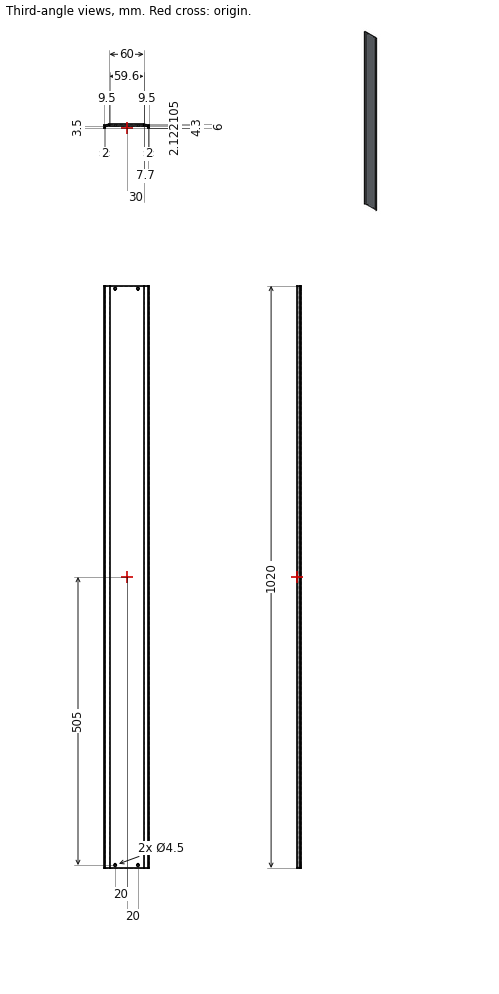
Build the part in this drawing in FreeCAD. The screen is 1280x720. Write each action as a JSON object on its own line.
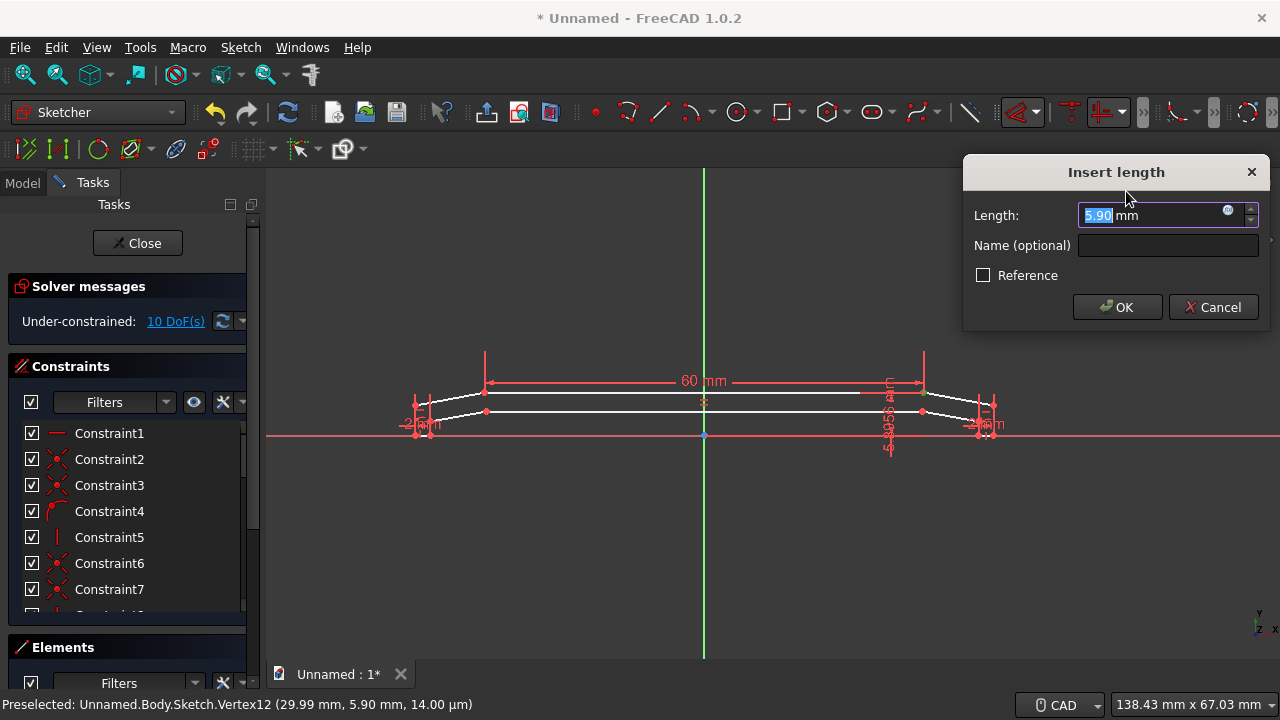
{"action": "type", "text": "6"}
{"action": "key", "text": "Return"}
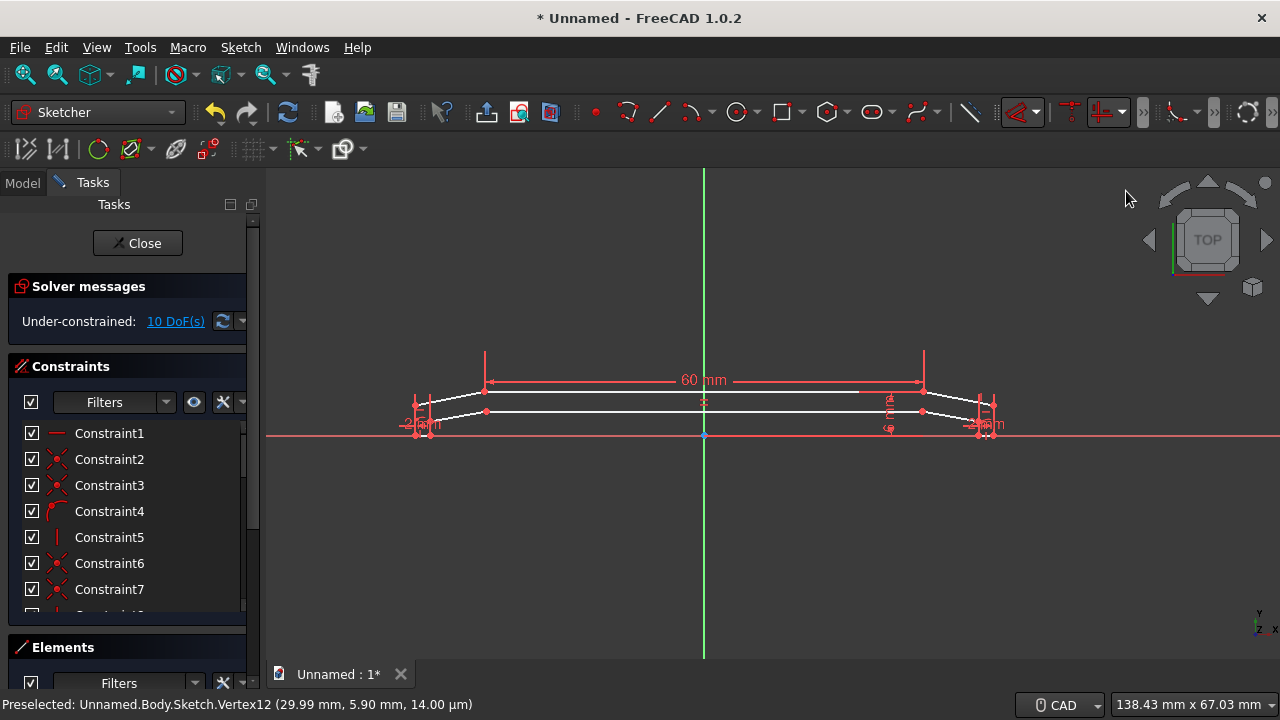
{"action": "scroll", "coordinate": [994, 427], "scroll_direction": "up", "scroll_amount": 3}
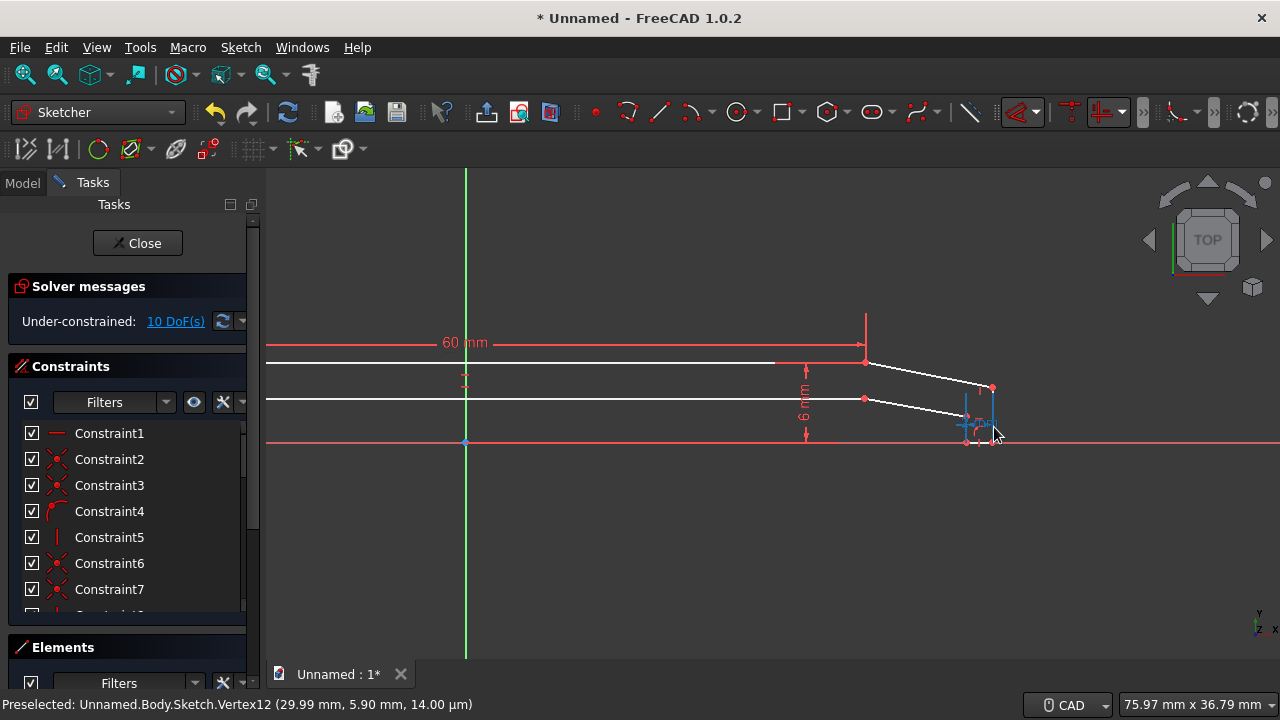
{"action": "left_click", "coordinate": [993, 404]}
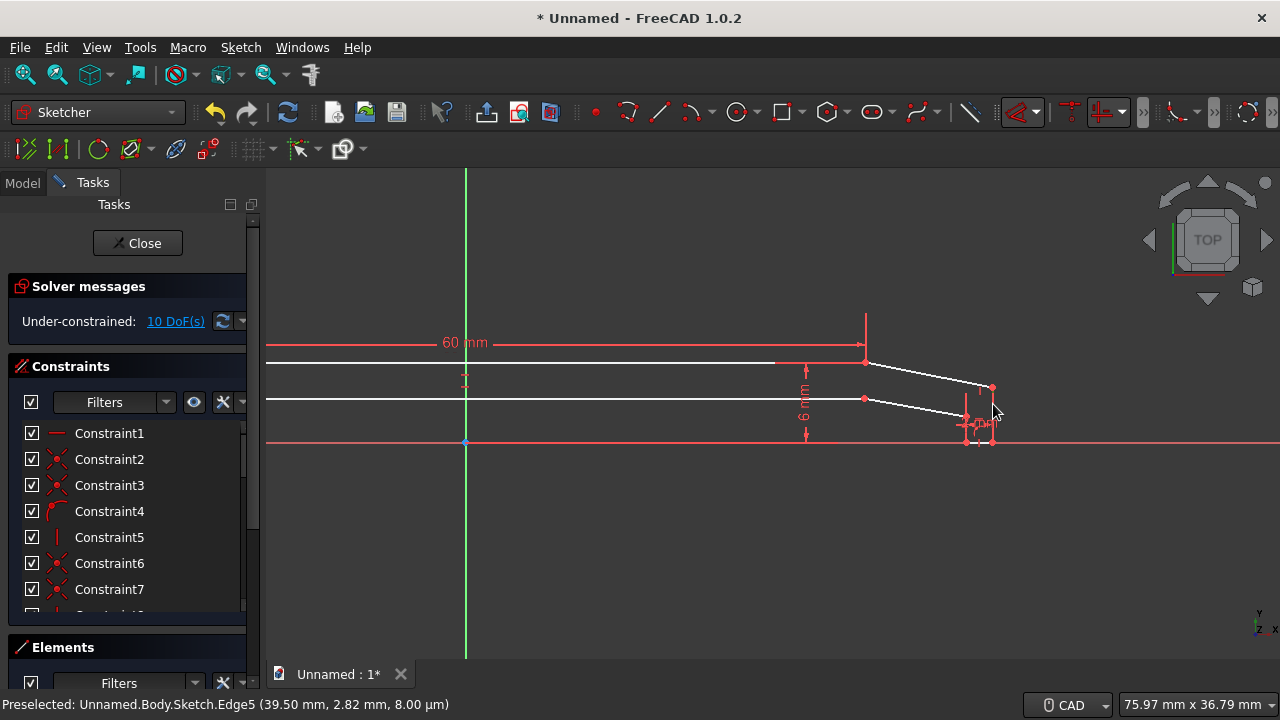
{"action": "left_click", "coordinate": [1038, 112]}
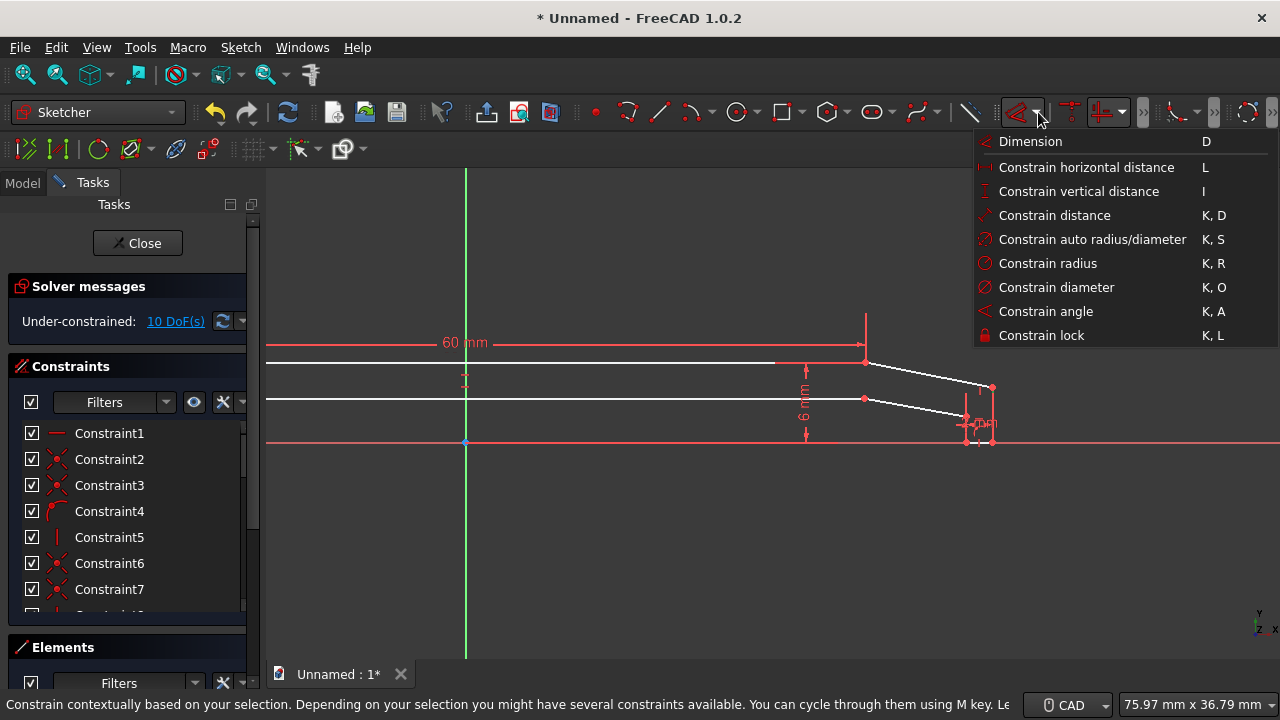
{"action": "left_click", "coordinate": [1126, 191]}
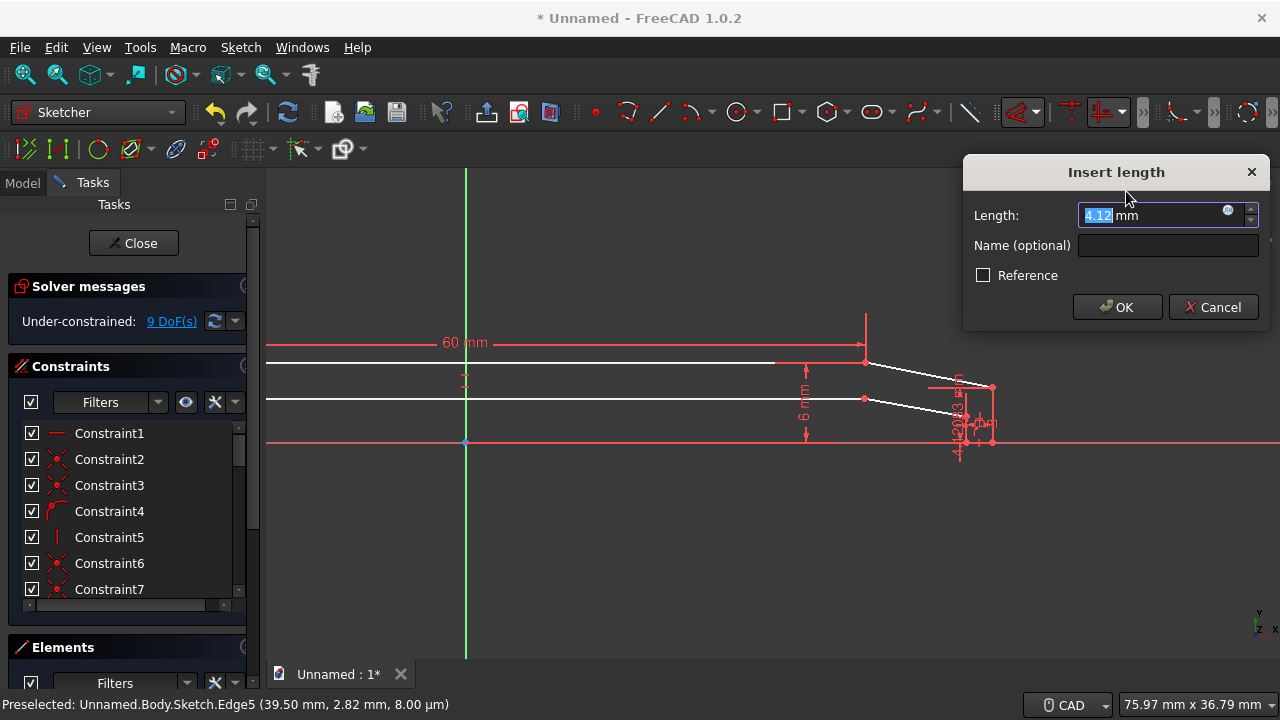
{"action": "type", "text": "4.3"}
{"action": "key", "text": "Return"}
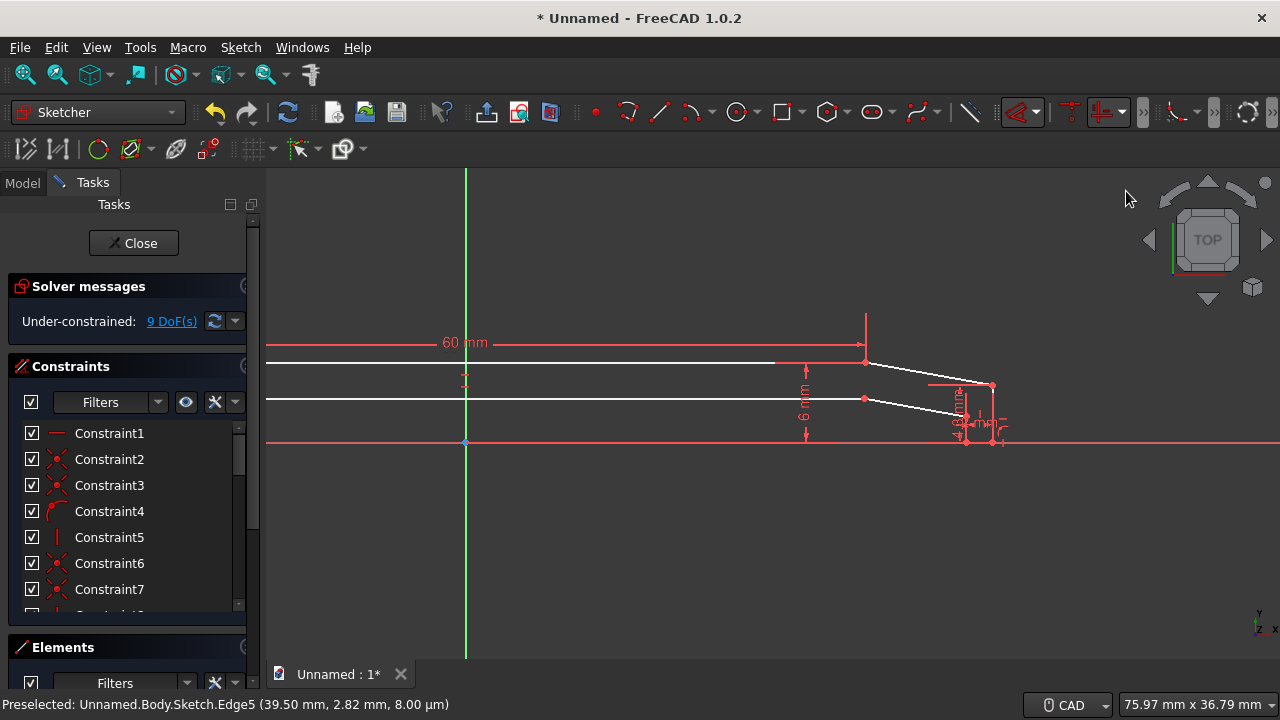
{"action": "scroll", "coordinate": [995, 427], "scroll_direction": "down", "scroll_amount": 3}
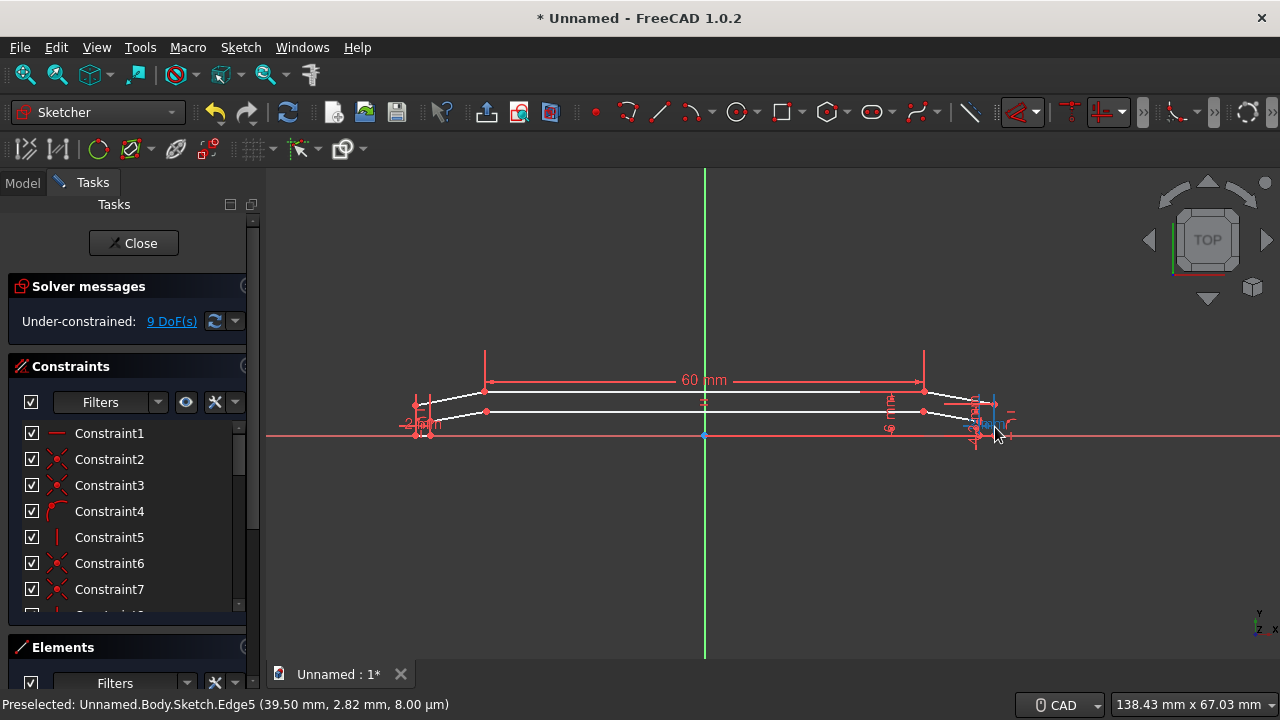
{"action": "scroll", "coordinate": [416, 415], "scroll_direction": "up", "scroll_amount": 3}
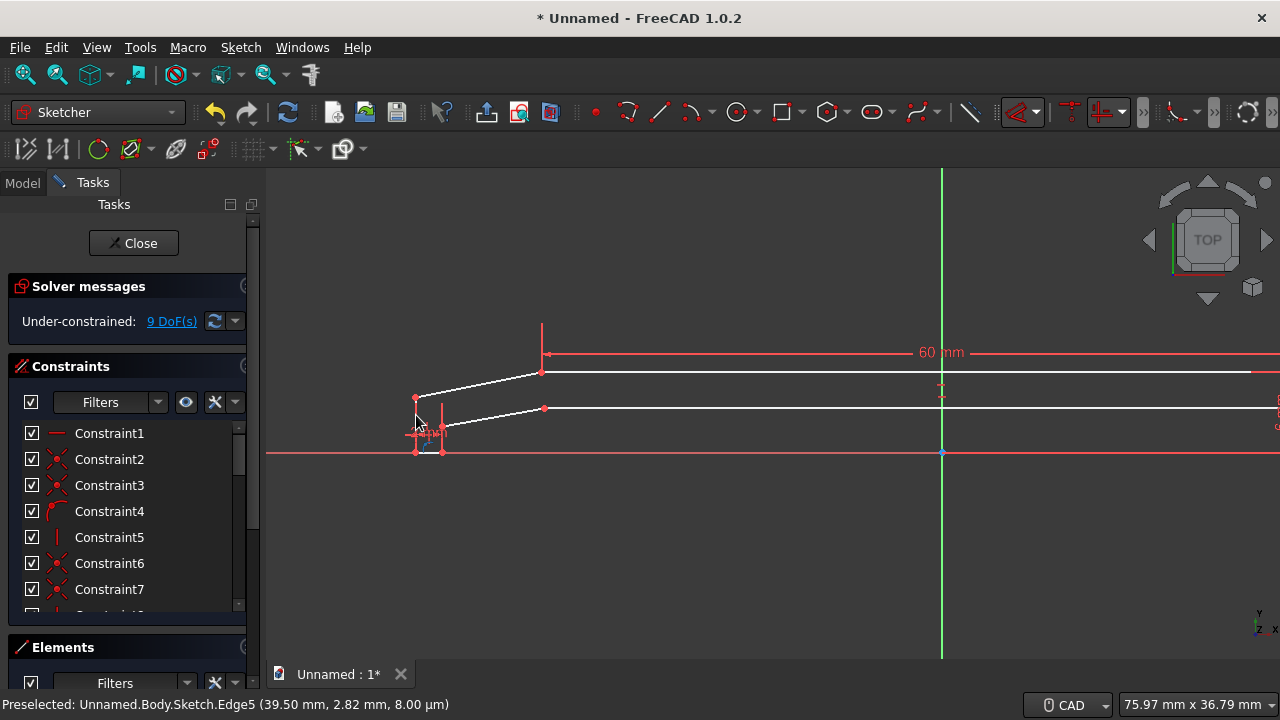
{"action": "left_click", "coordinate": [416, 414]}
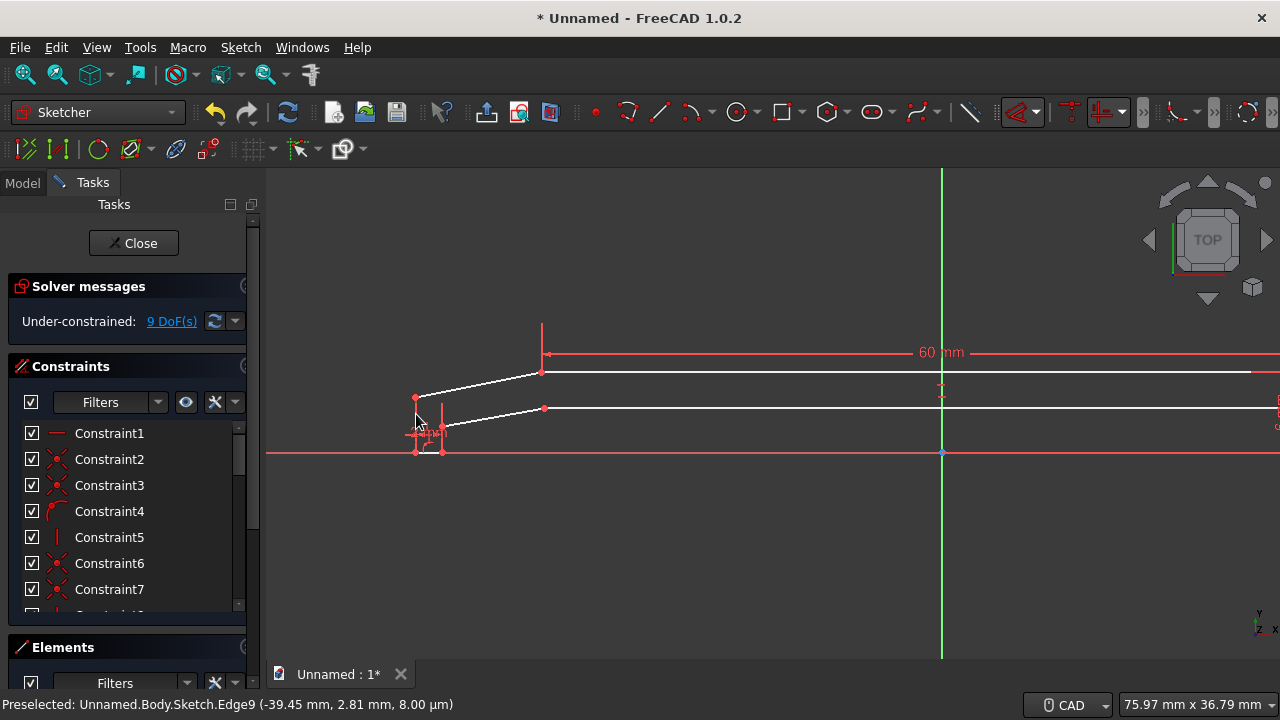
{"action": "left_click", "coordinate": [1038, 112]}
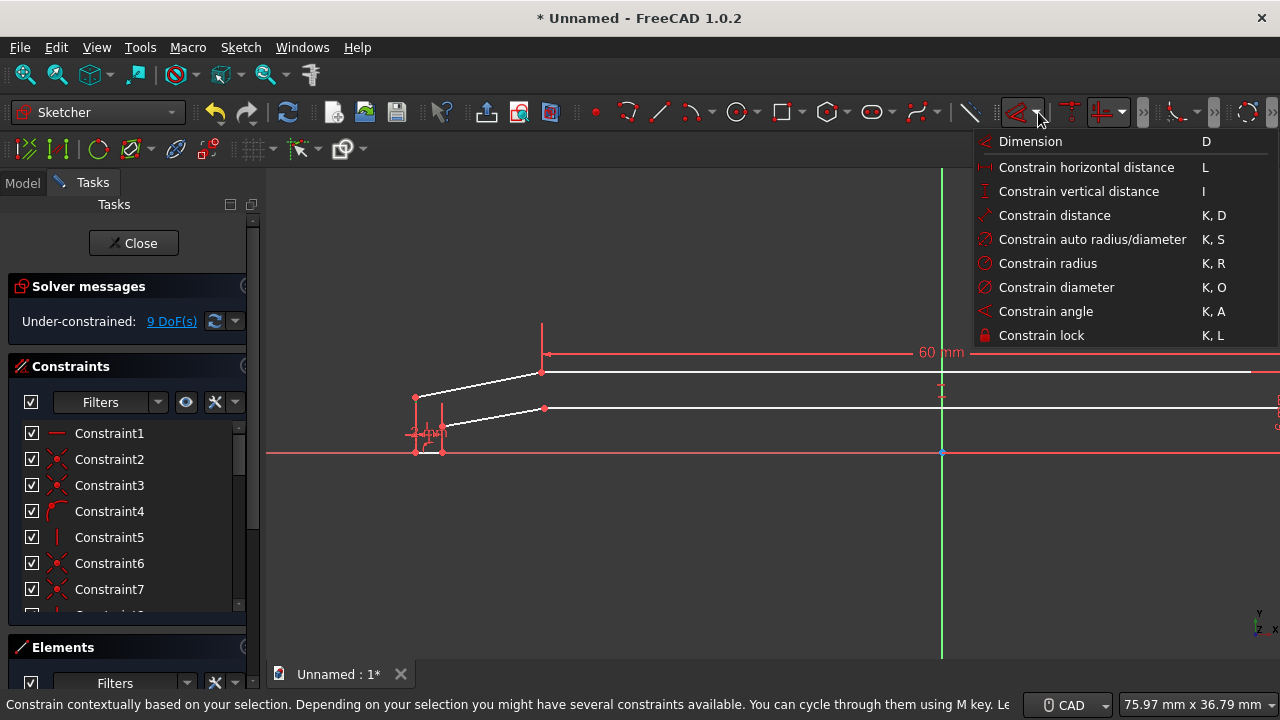
{"action": "left_click", "coordinate": [1126, 191]}